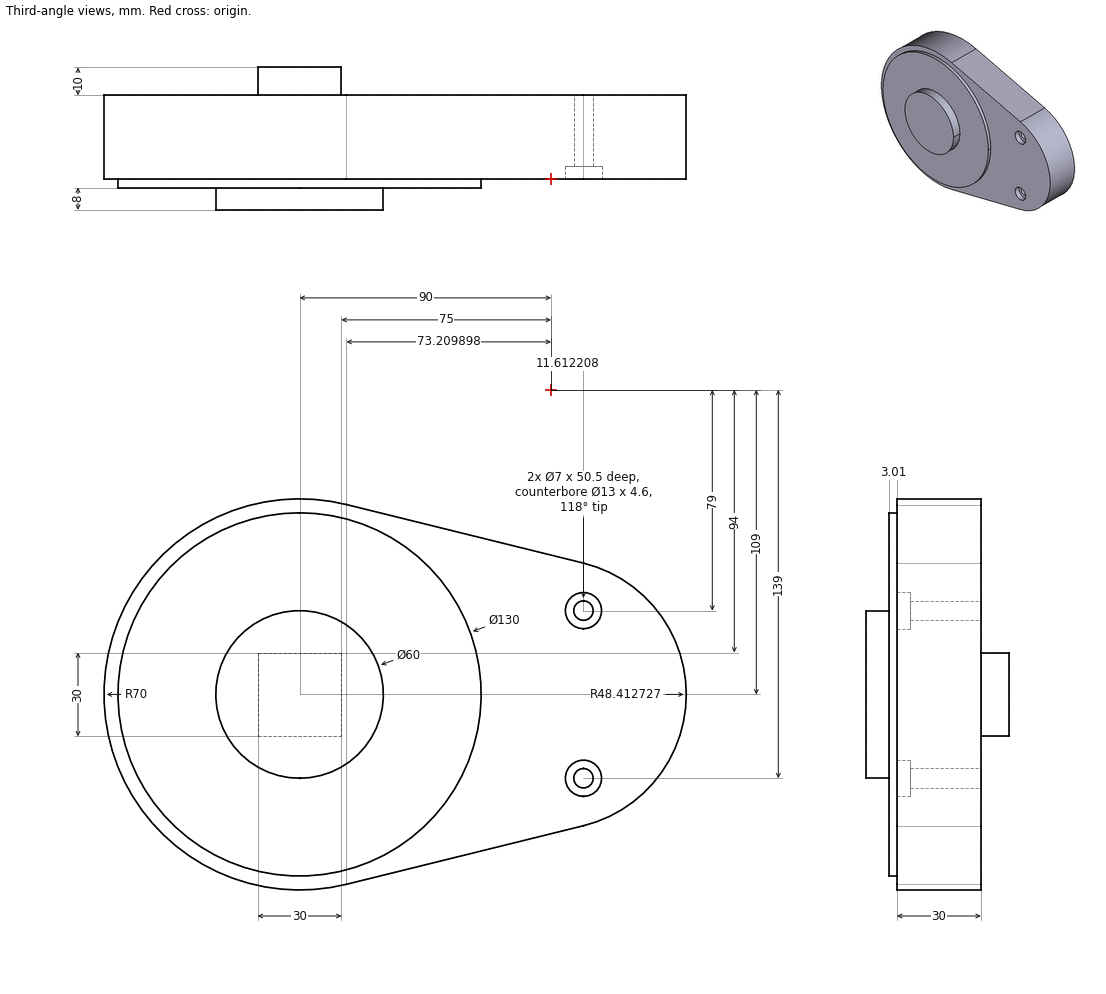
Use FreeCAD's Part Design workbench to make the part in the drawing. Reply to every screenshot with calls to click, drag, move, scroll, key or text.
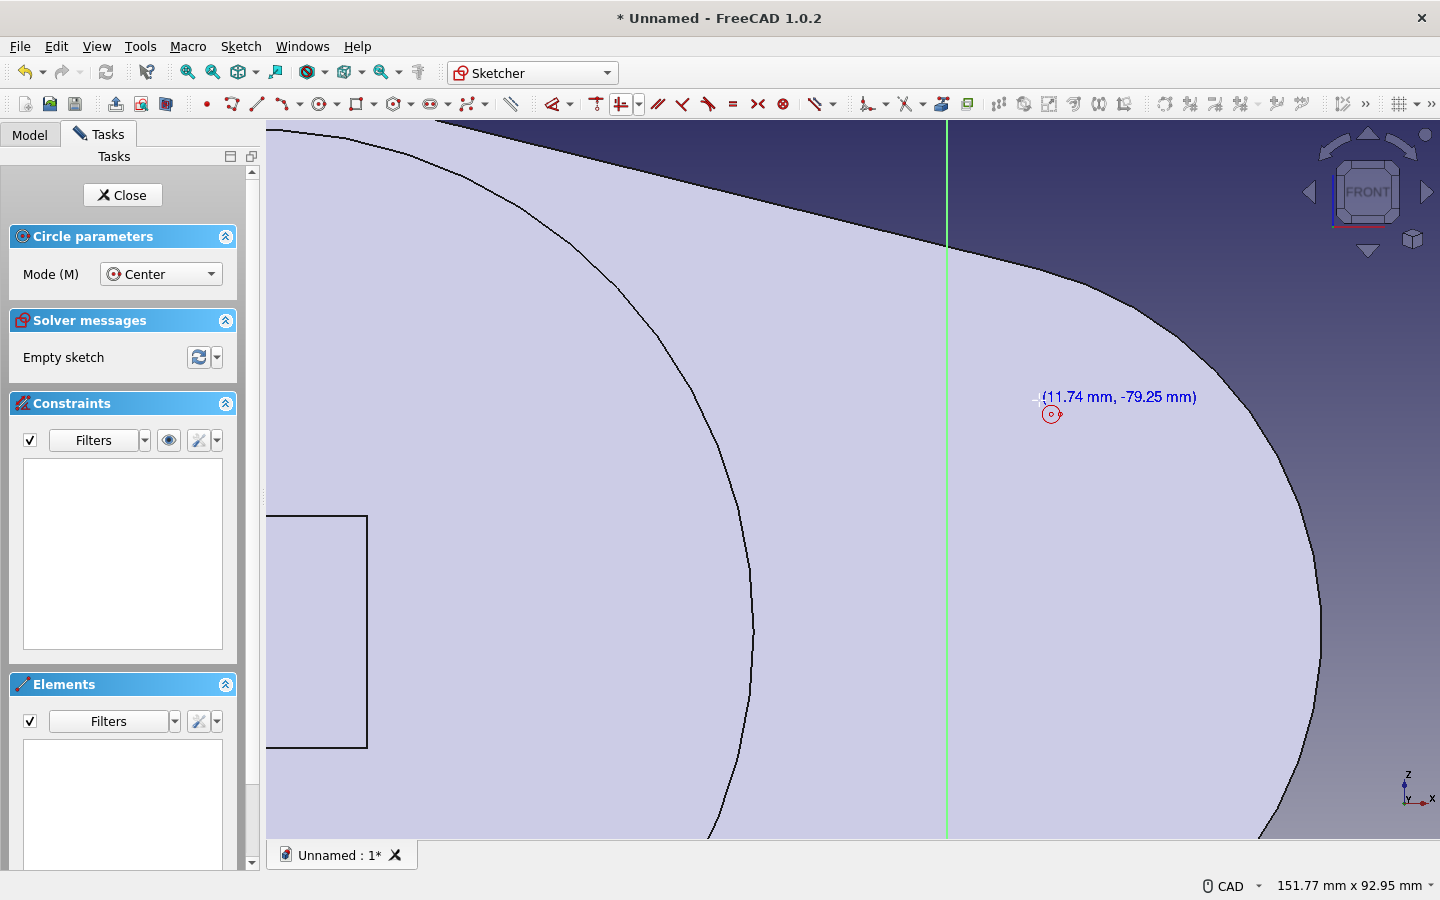
click(1037, 400)
click(1056, 381)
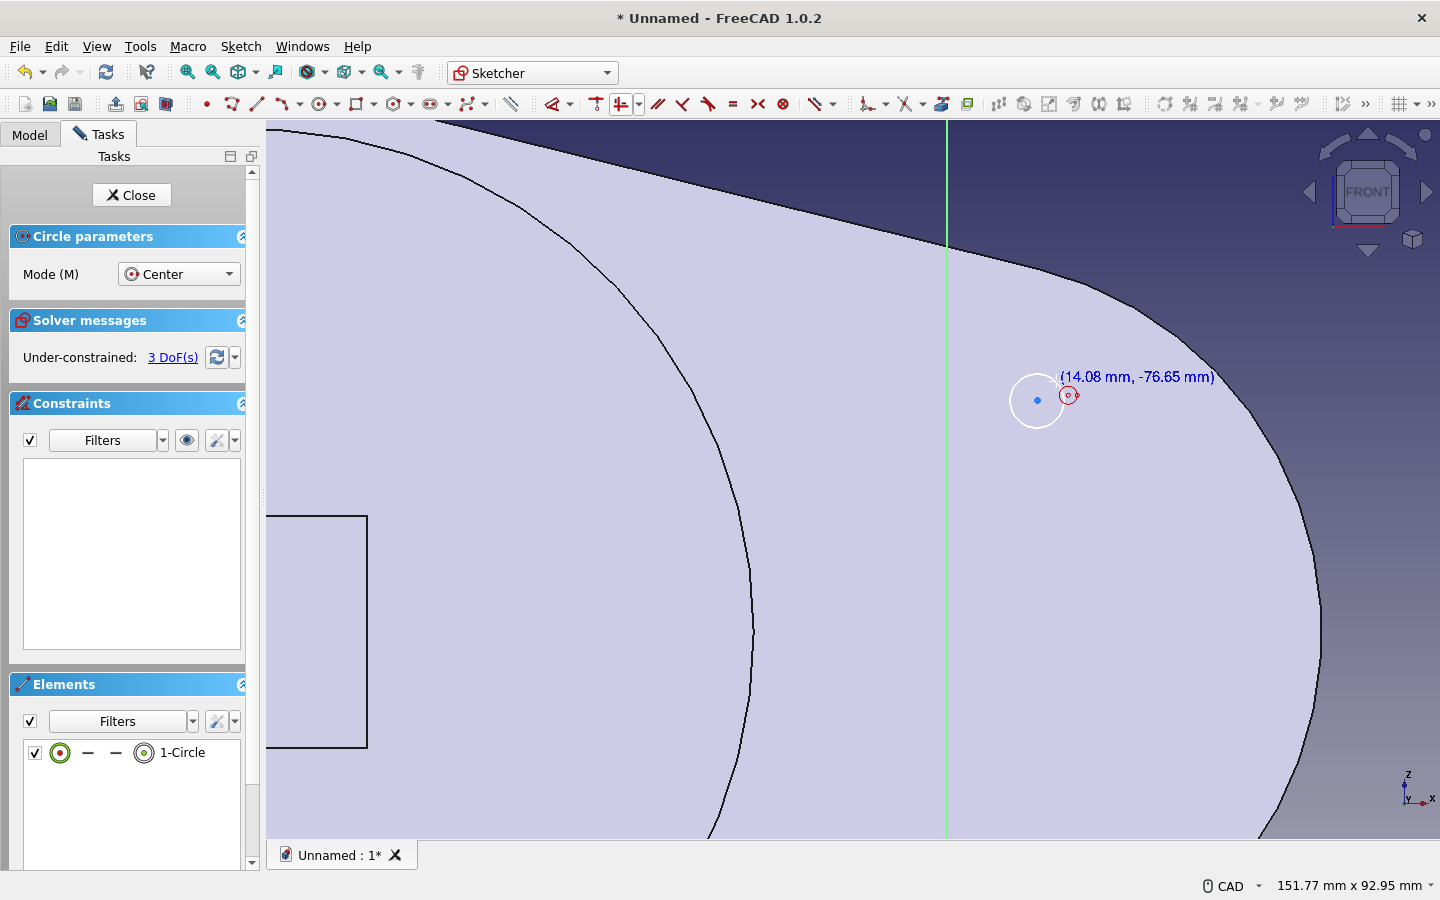
scroll(604, 593, down, 4)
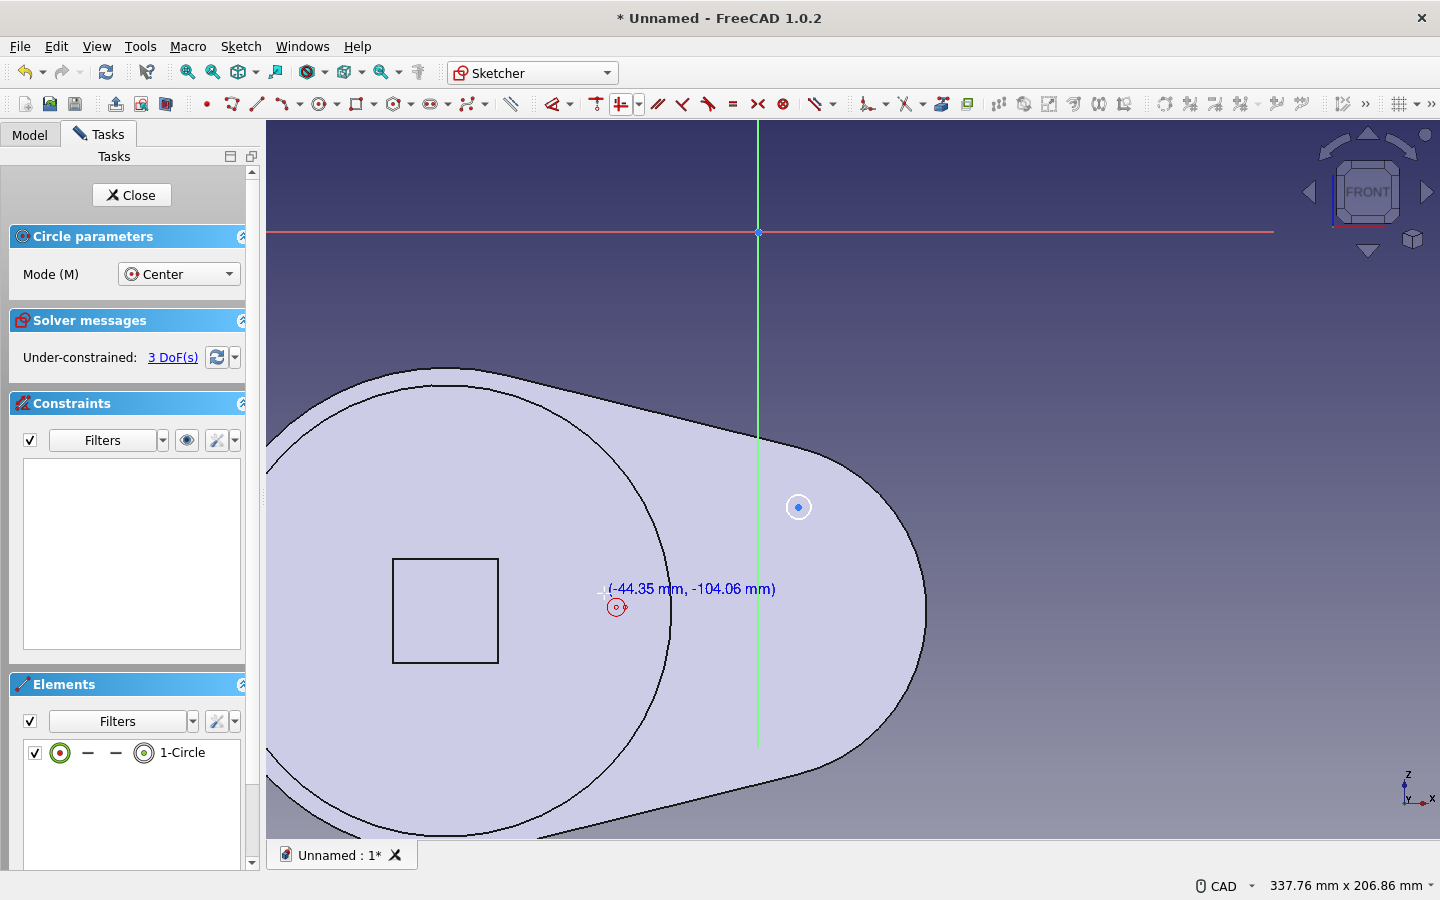
scroll(799, 715, up, 4)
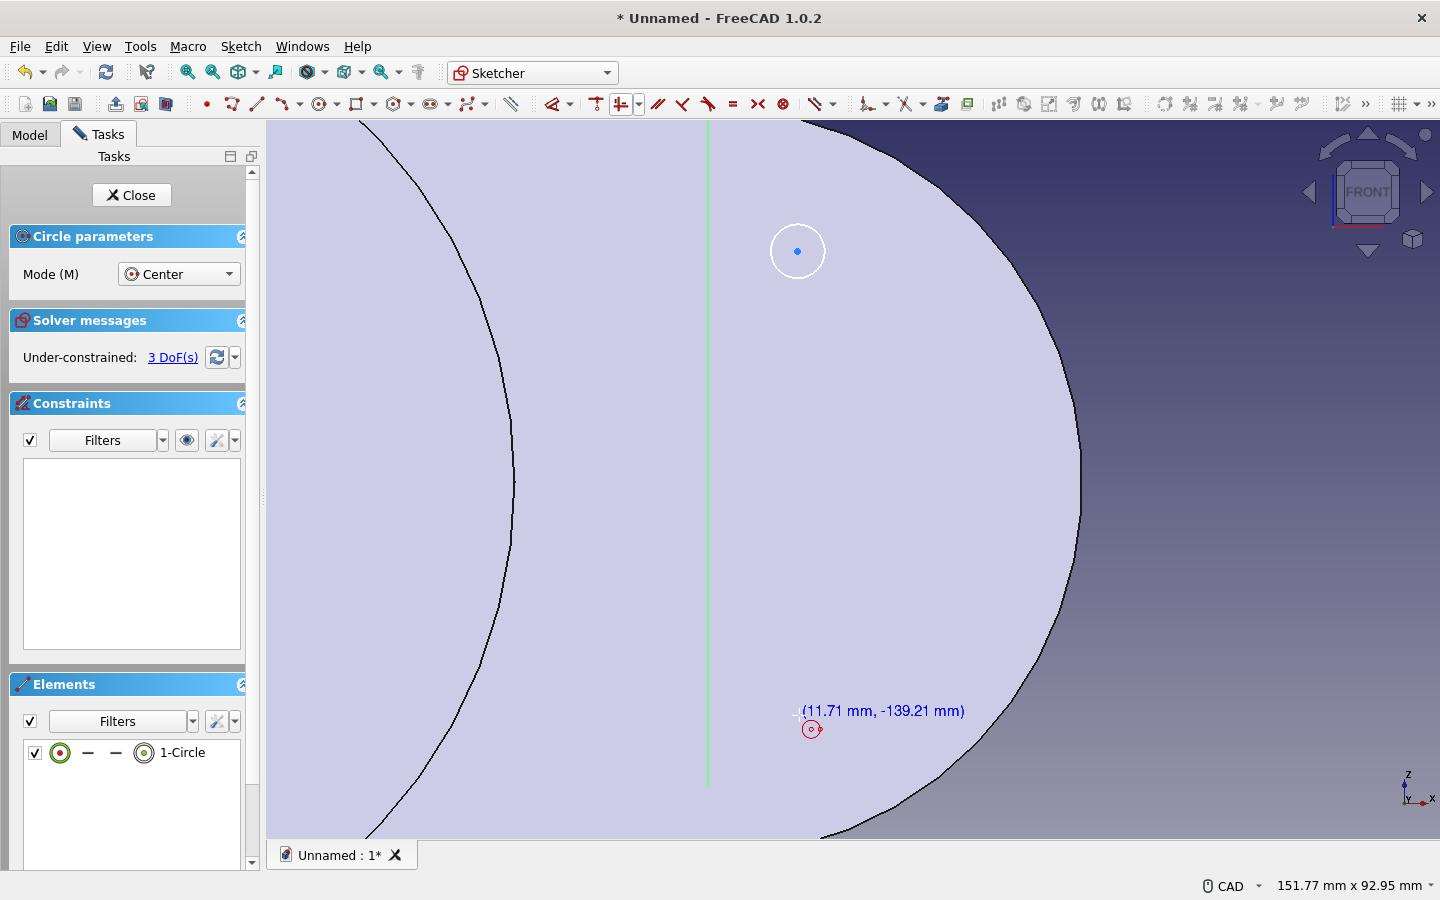
click(798, 715)
click(817, 695)
key(Escape)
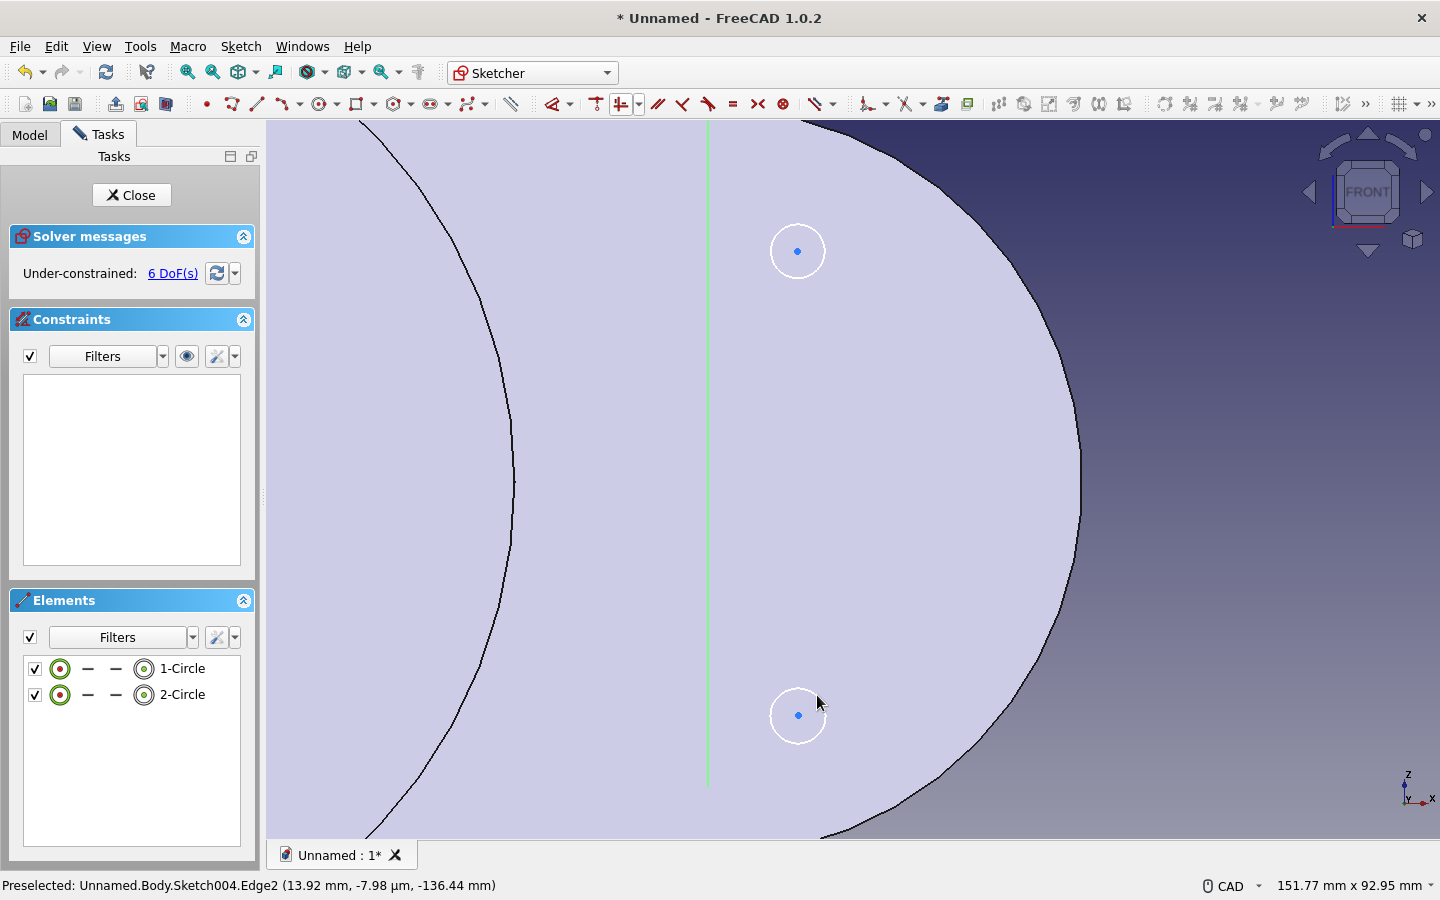
click(817, 232)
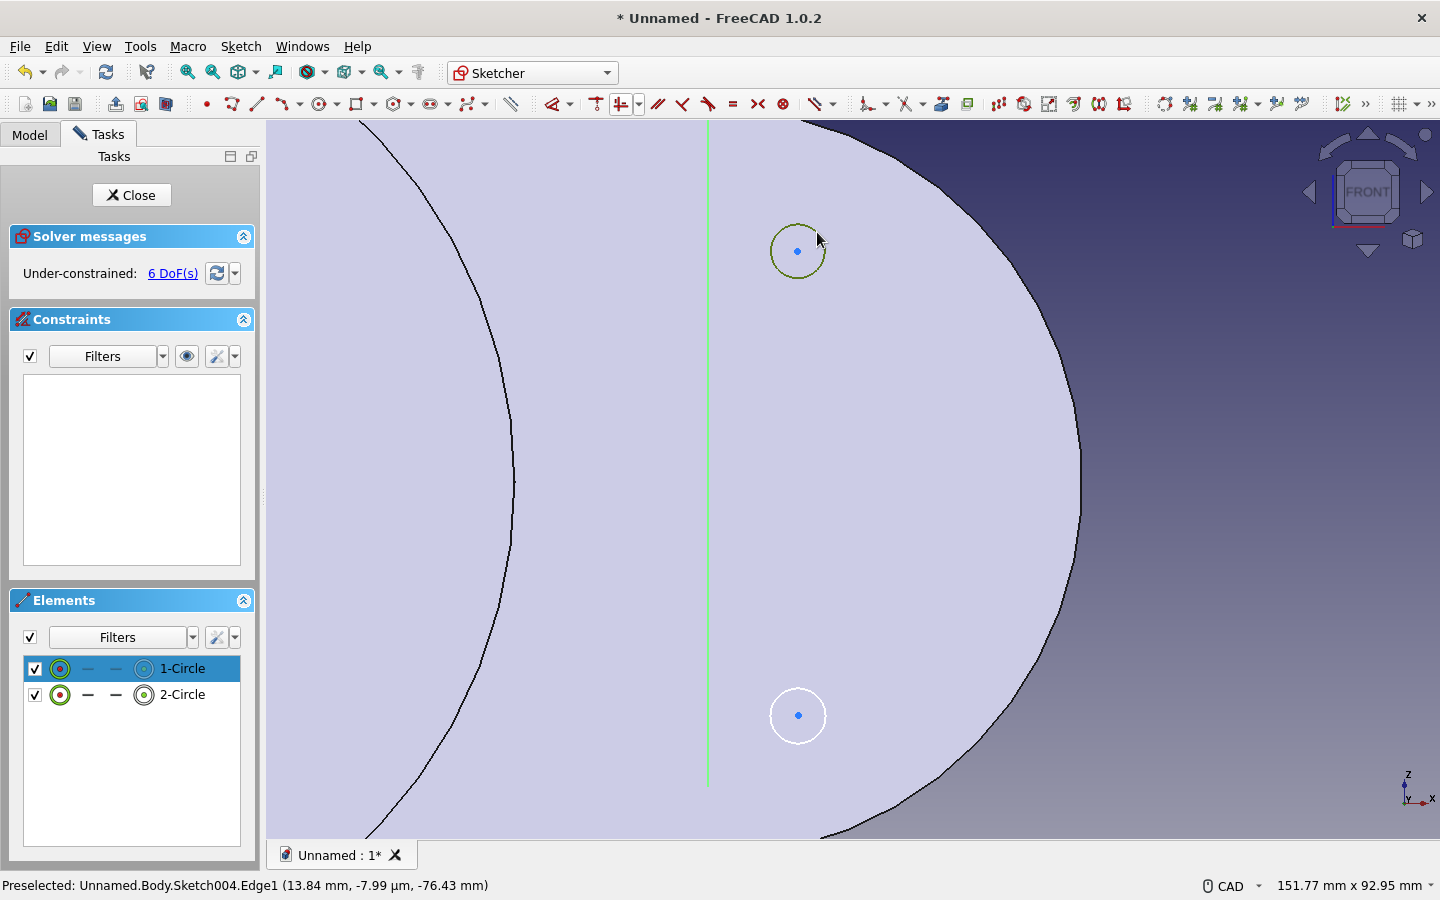
click(817, 696)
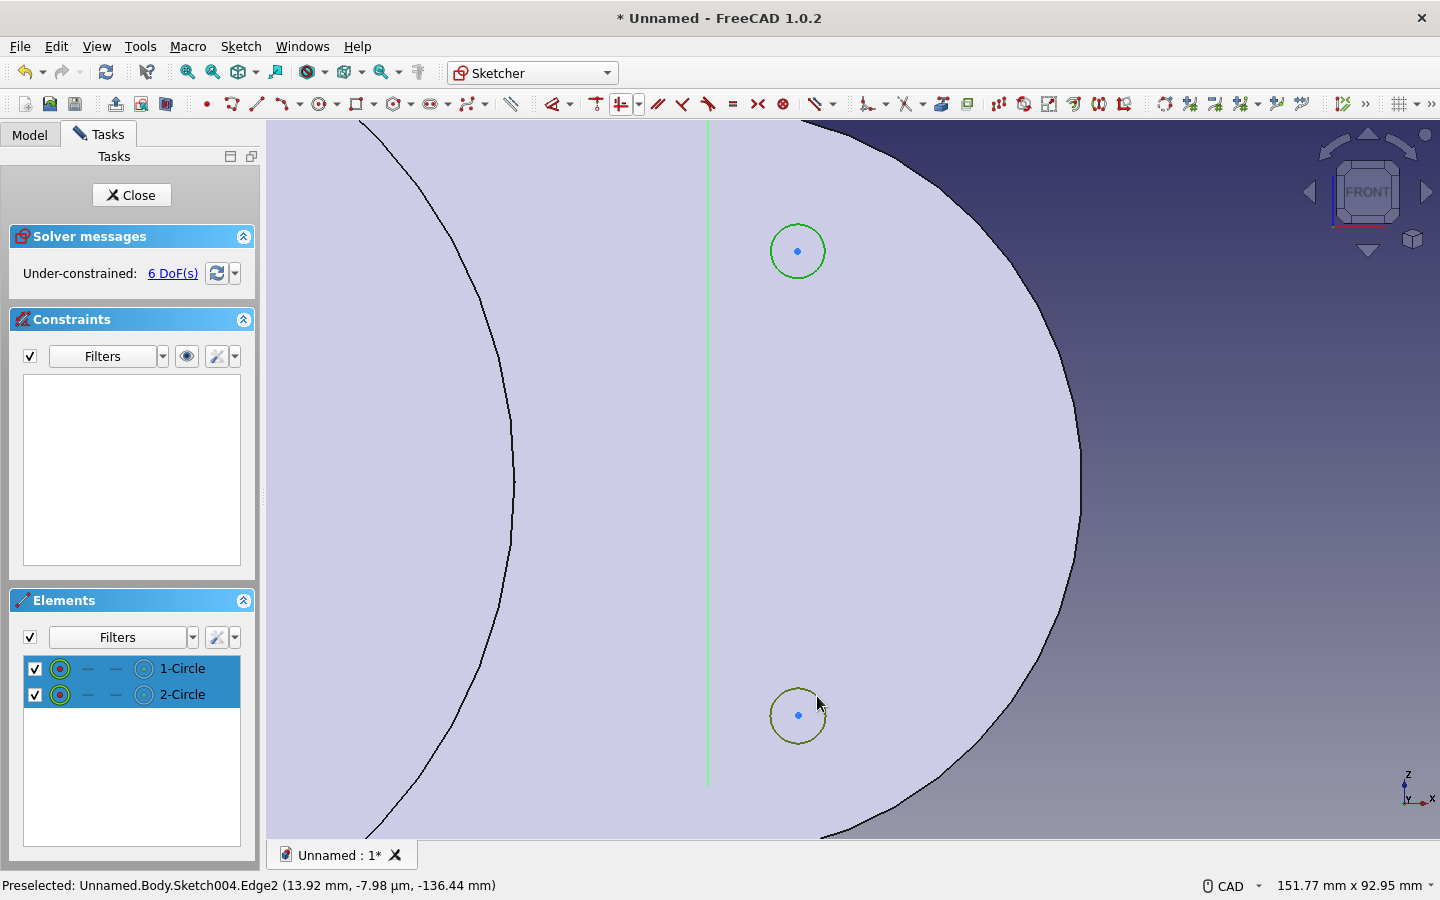
key(e)